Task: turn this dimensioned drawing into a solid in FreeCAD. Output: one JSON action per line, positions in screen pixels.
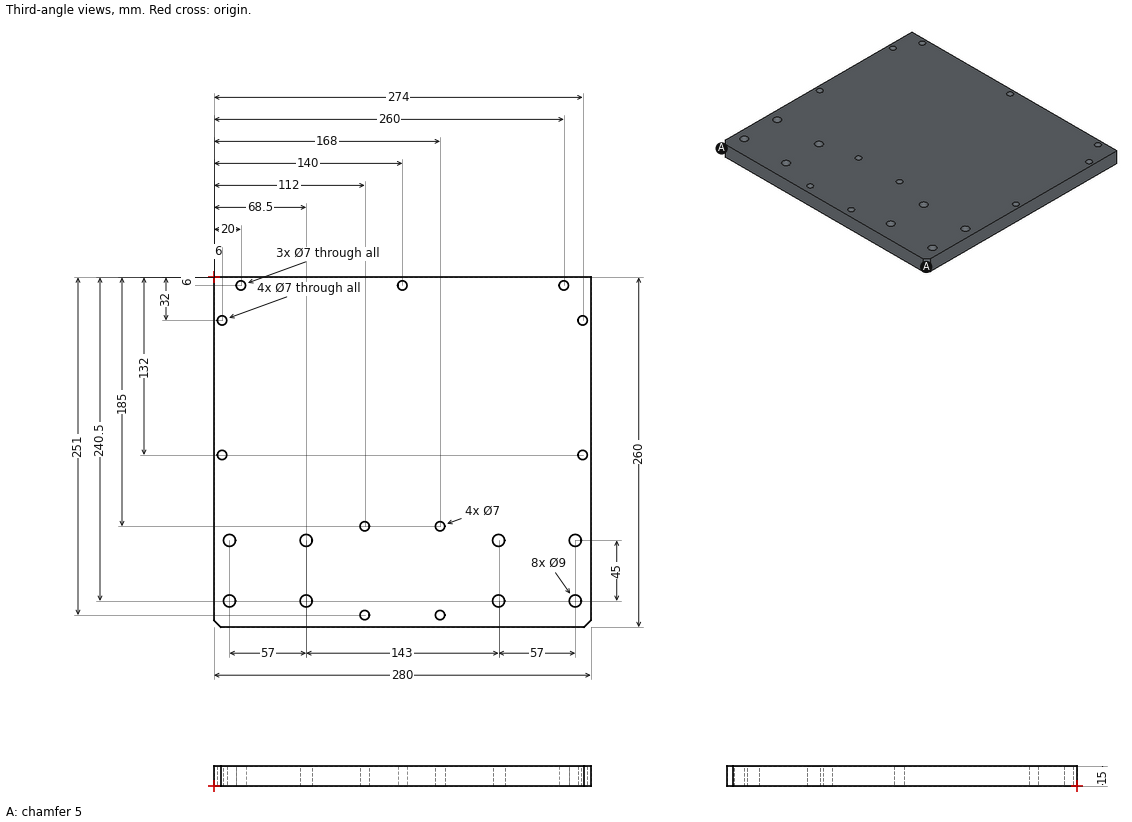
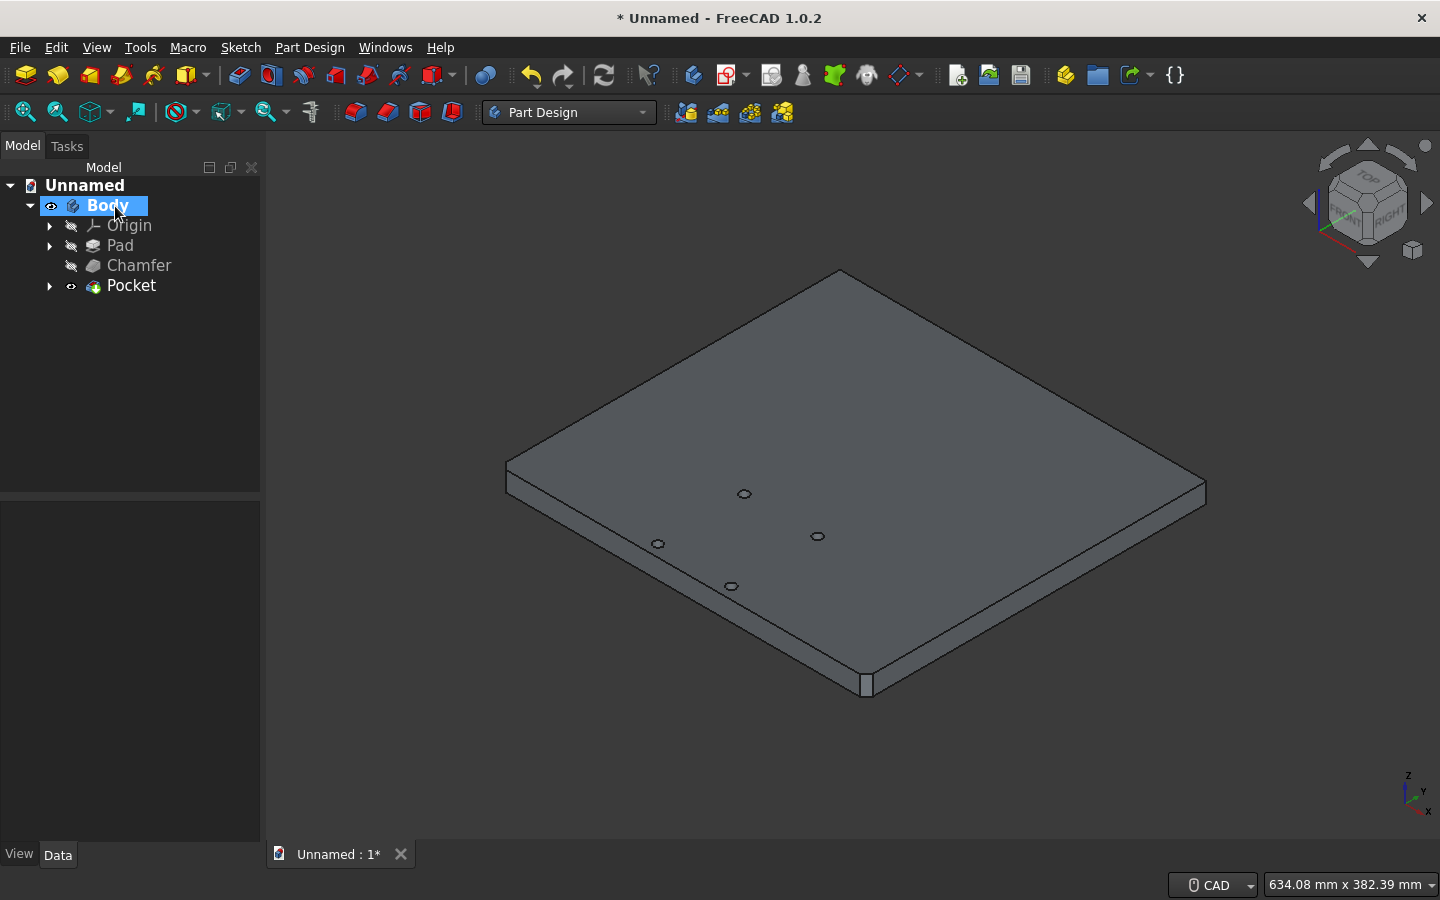
{"action": "left_click", "coordinate": [902, 445]}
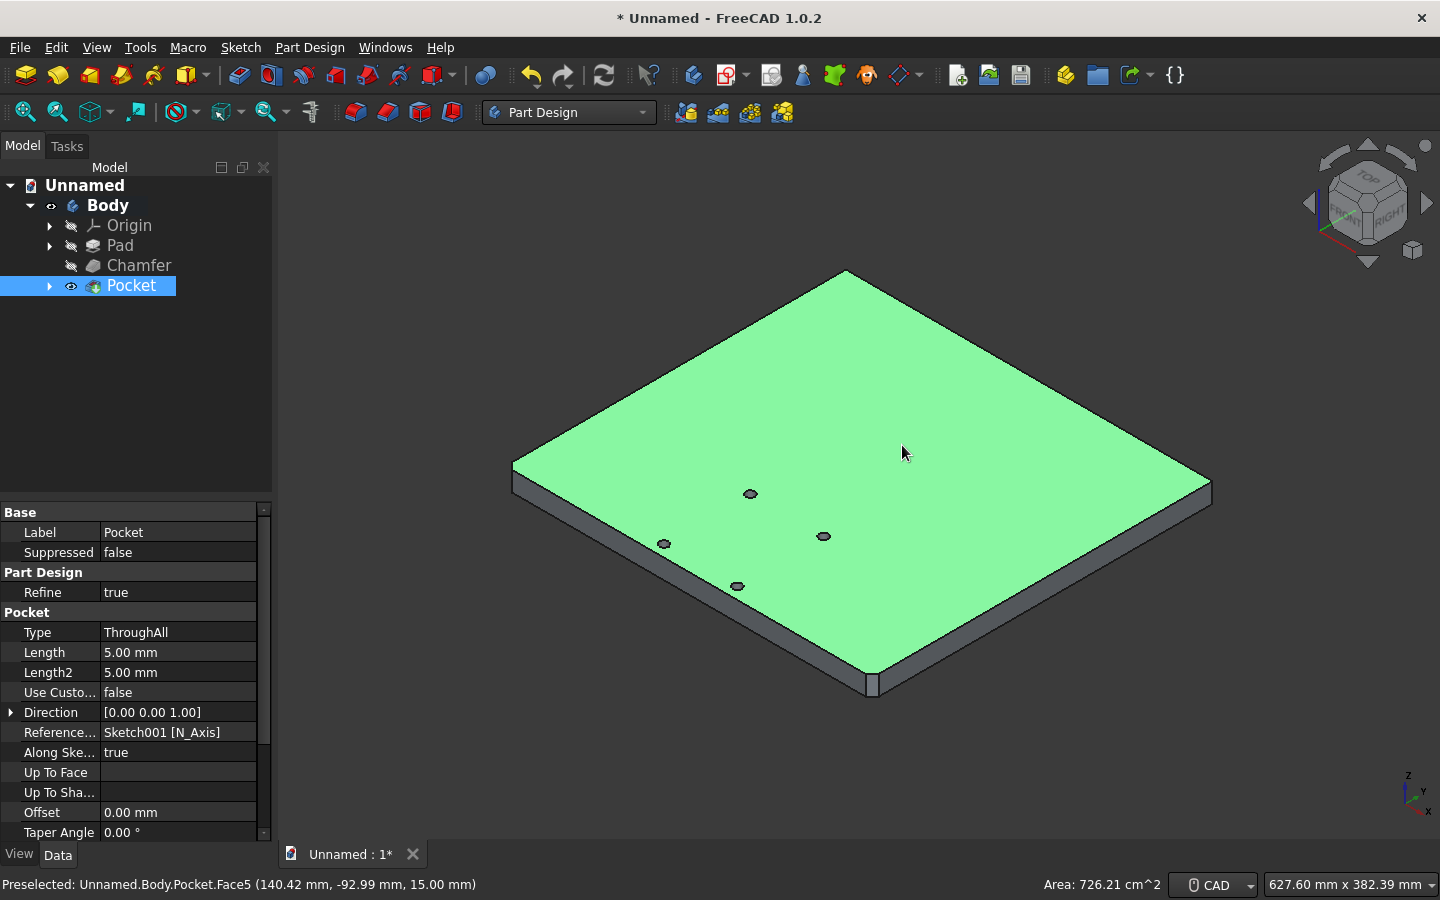
{"action": "left_click", "coordinate": [726, 76]}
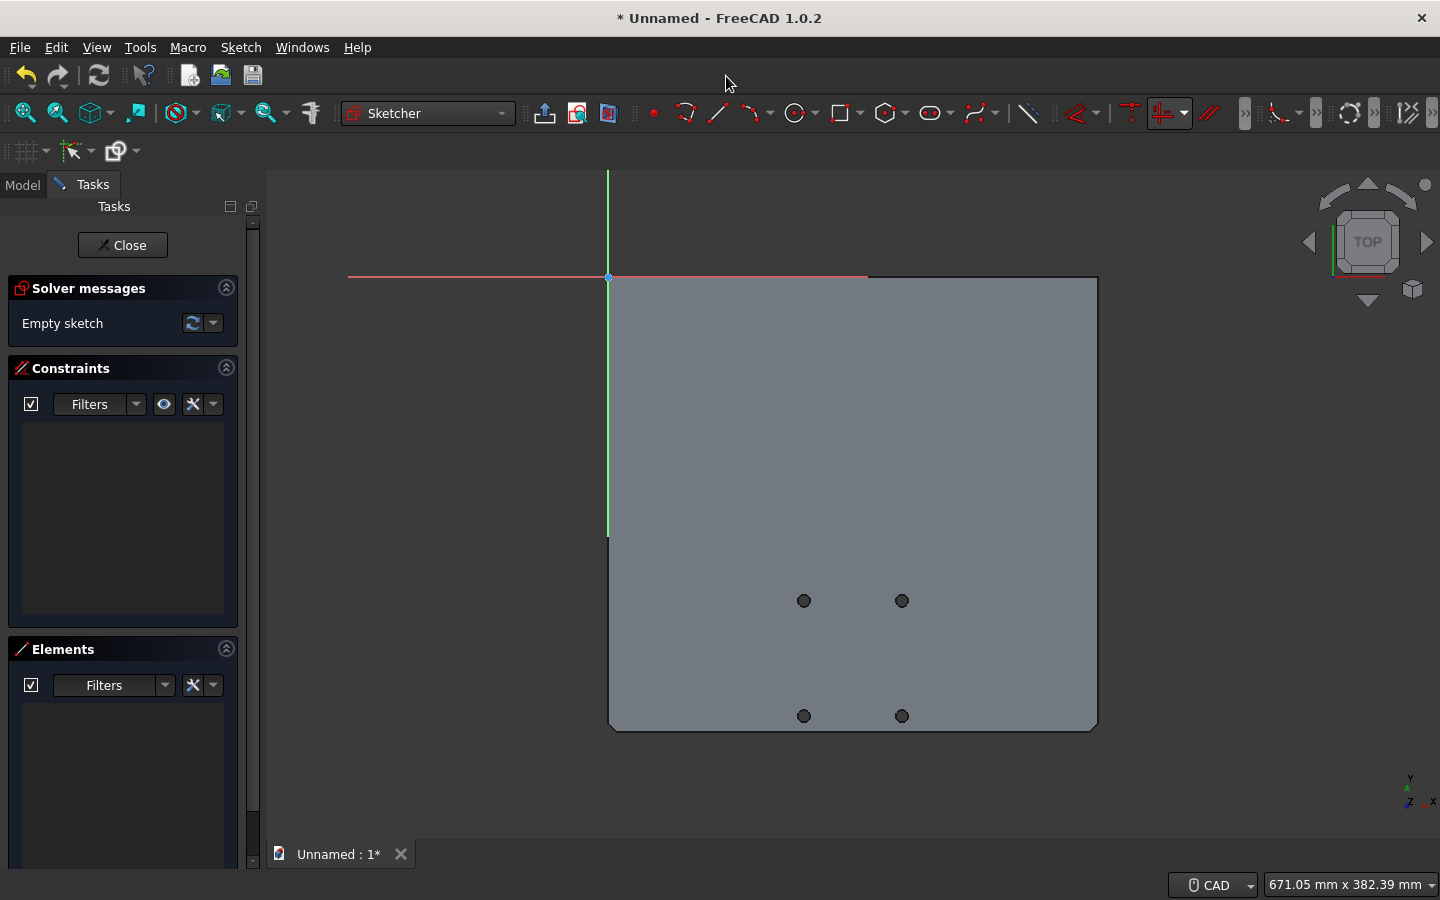
{"action": "scroll", "coordinate": [948, 198], "scroll_direction": "up", "scroll_amount": 2}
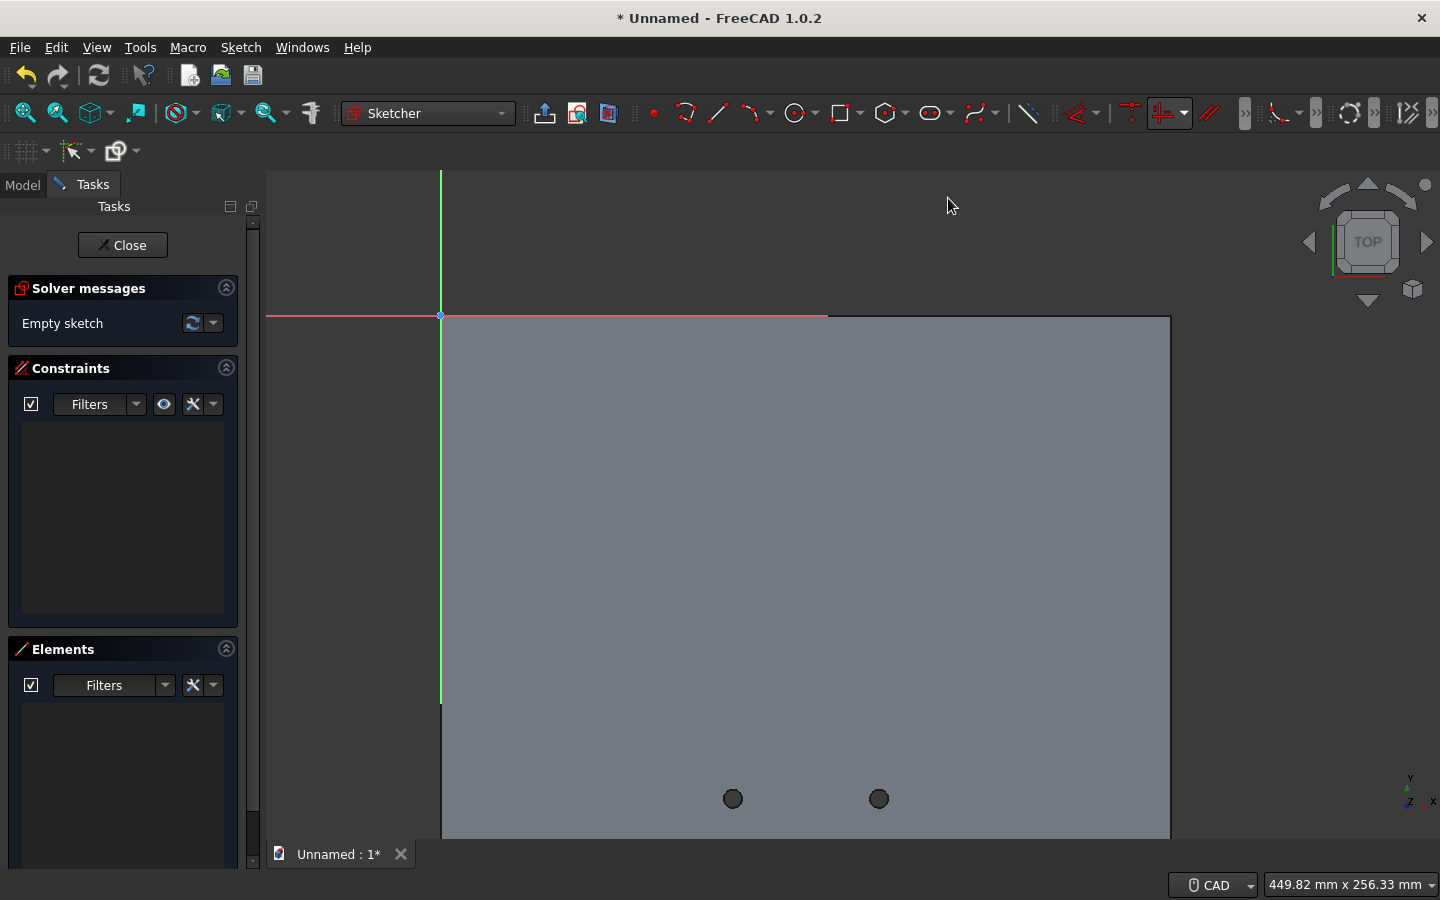
{"action": "left_click", "coordinate": [796, 114]}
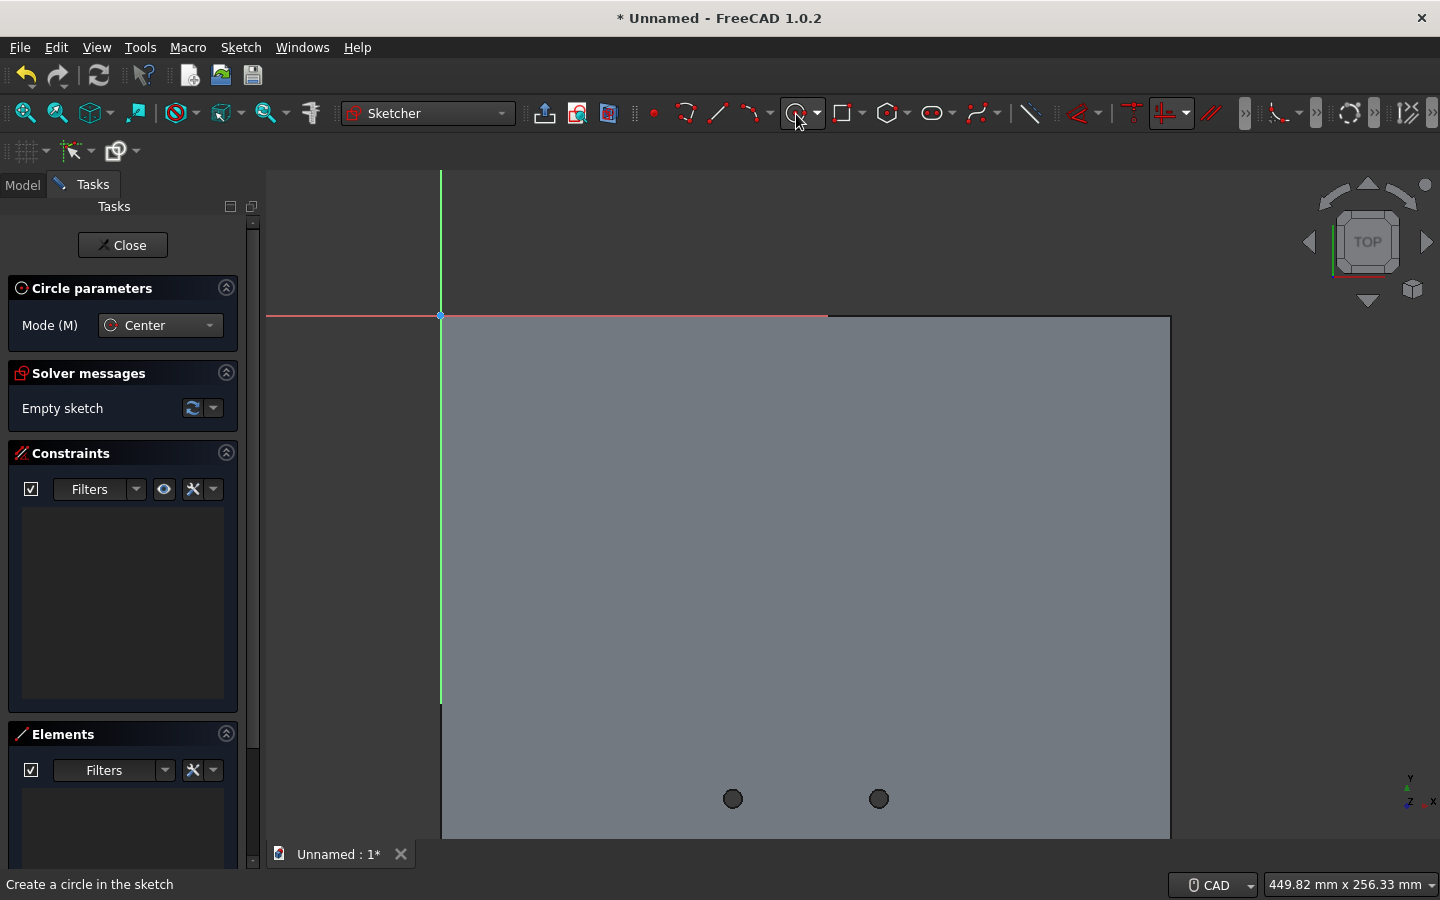
{"action": "scroll", "coordinate": [493, 332], "scroll_direction": "up", "scroll_amount": 5}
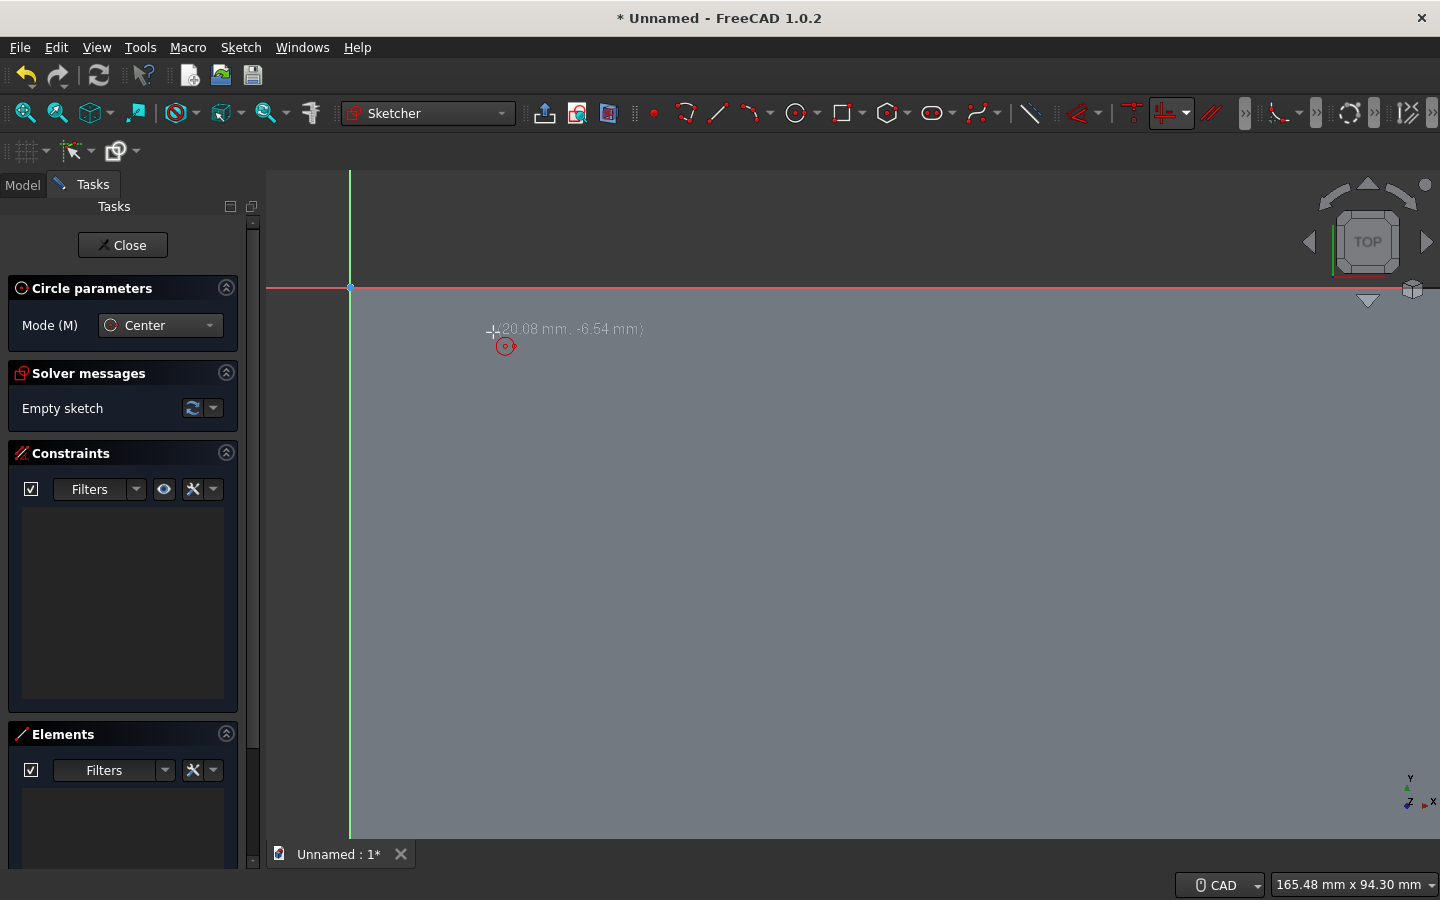
{"action": "left_click", "coordinate": [492, 330]}
{"action": "mouse_move", "coordinate": [510, 313]}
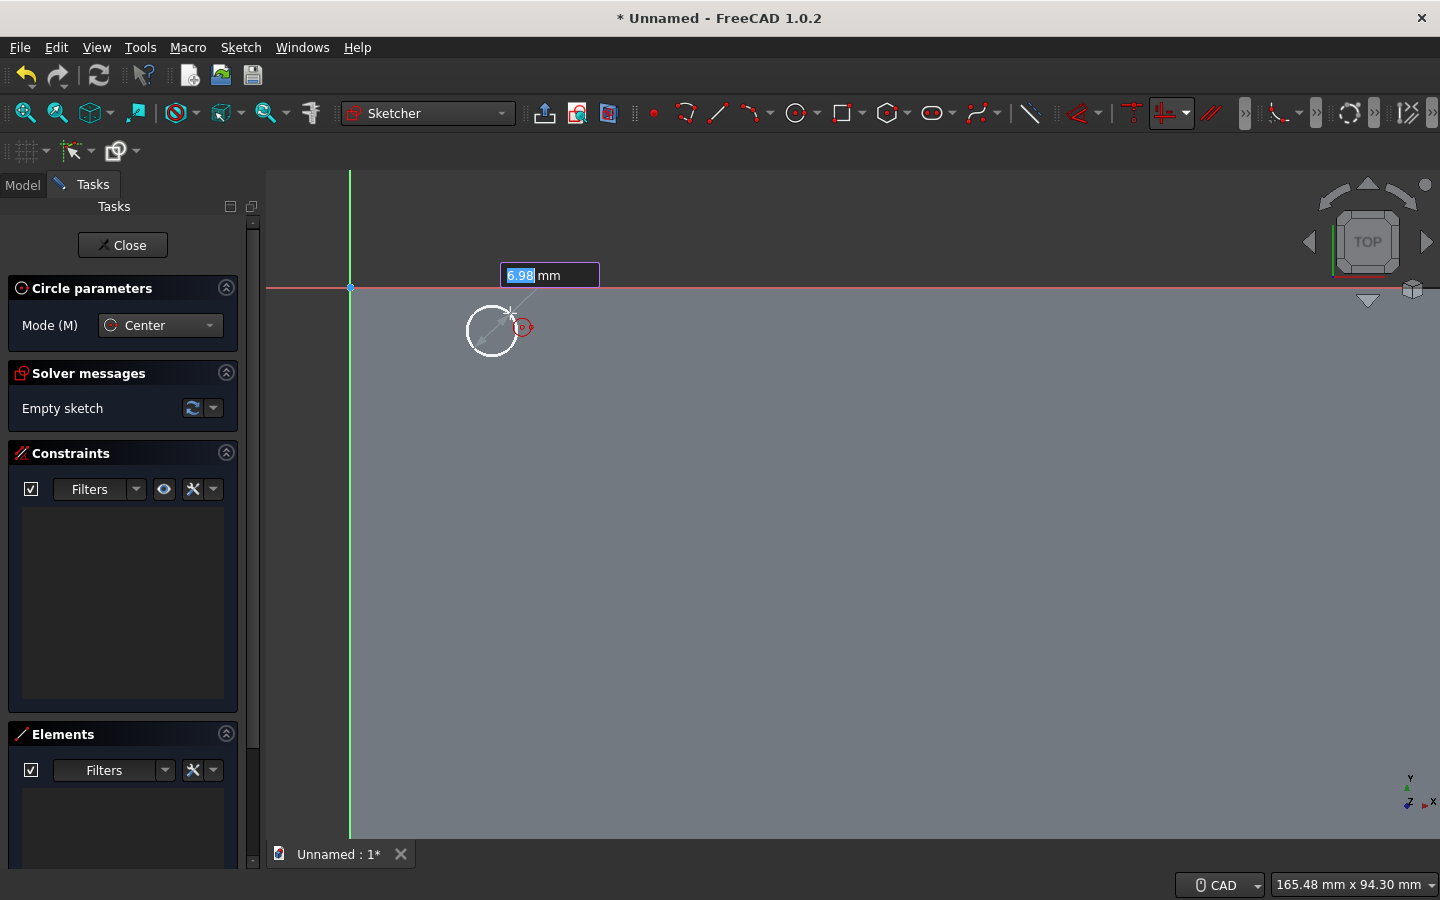
{"action": "type", "text": "7"}
{"action": "key", "text": "Return"}